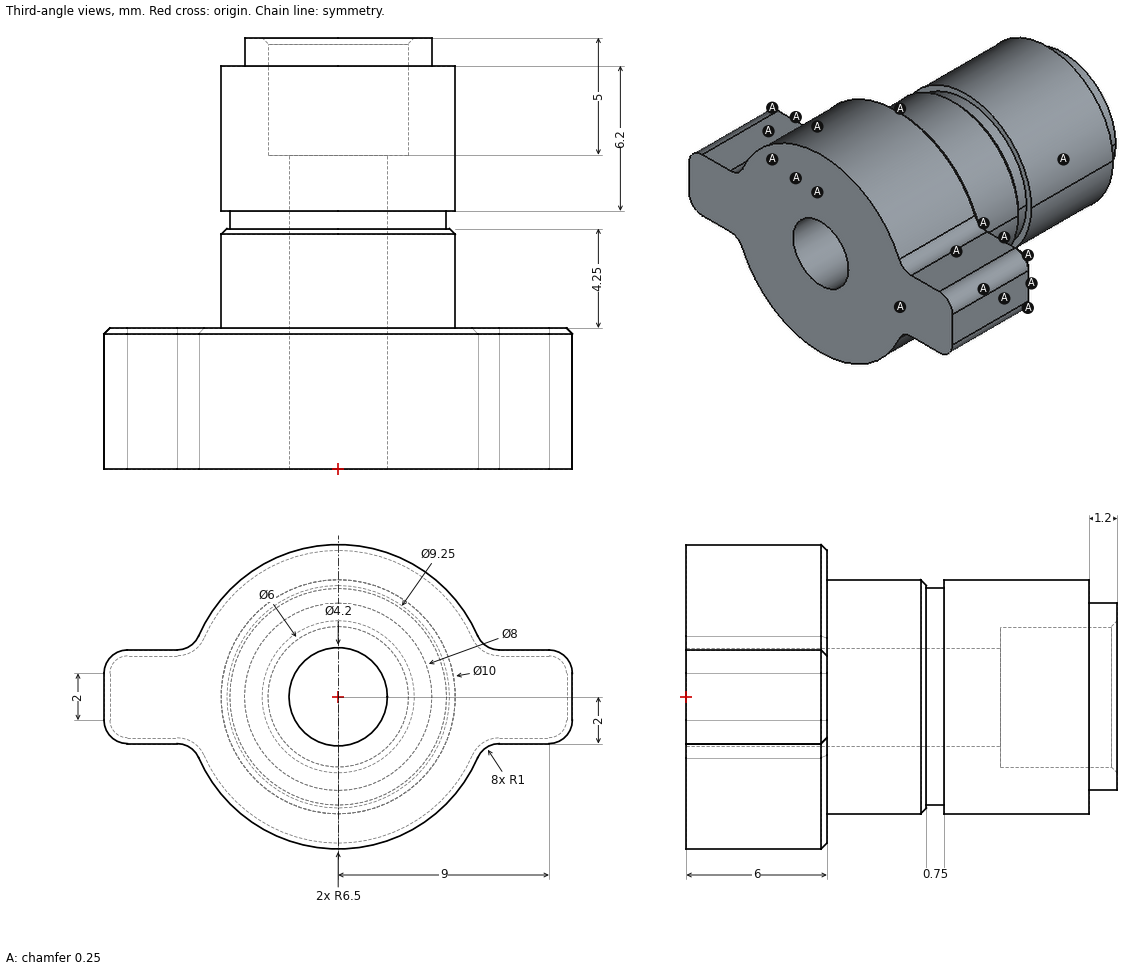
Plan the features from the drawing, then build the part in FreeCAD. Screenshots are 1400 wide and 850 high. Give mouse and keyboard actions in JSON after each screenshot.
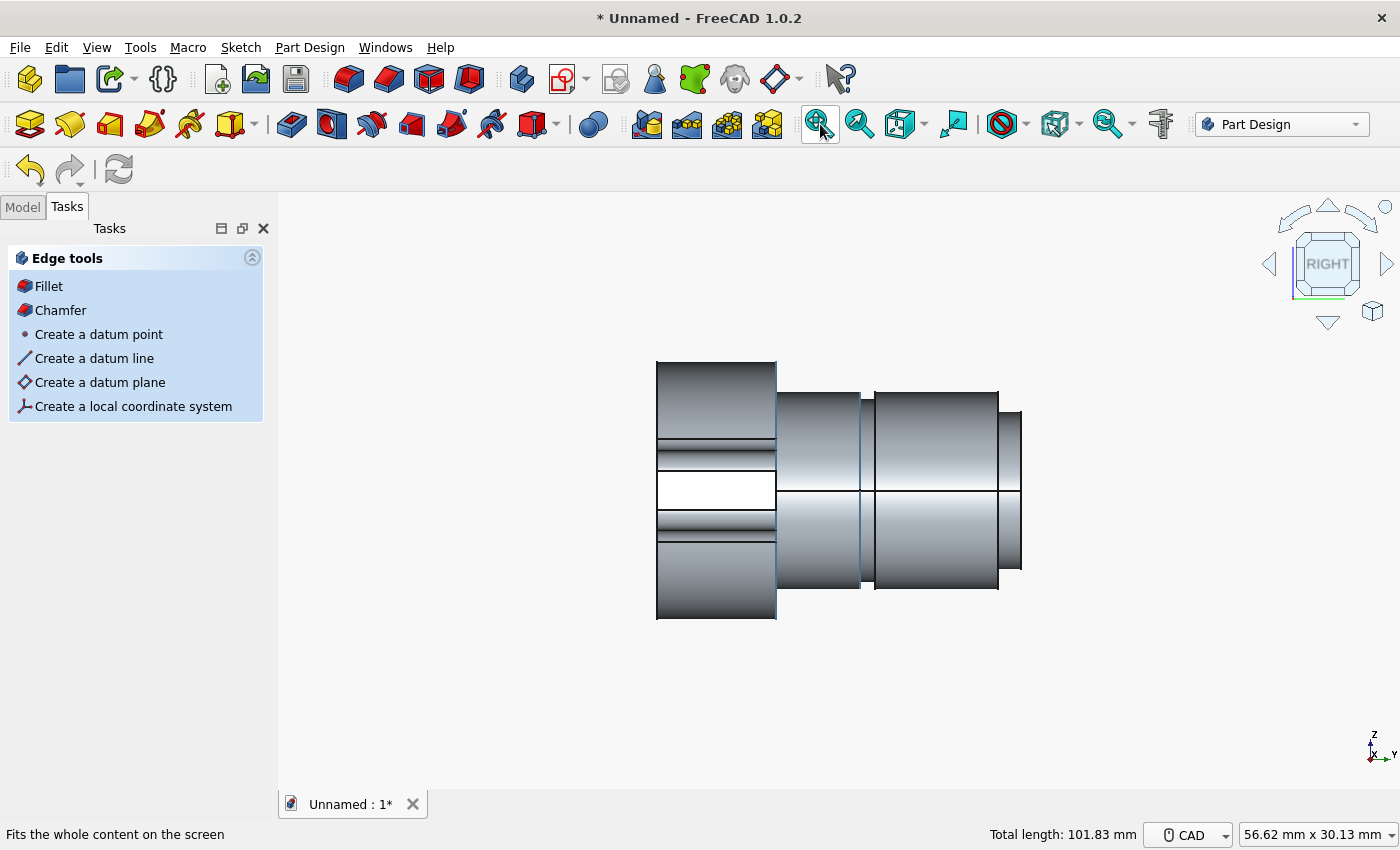
{"action": "left_click", "coordinate": [776, 490], "text": "ctrl"}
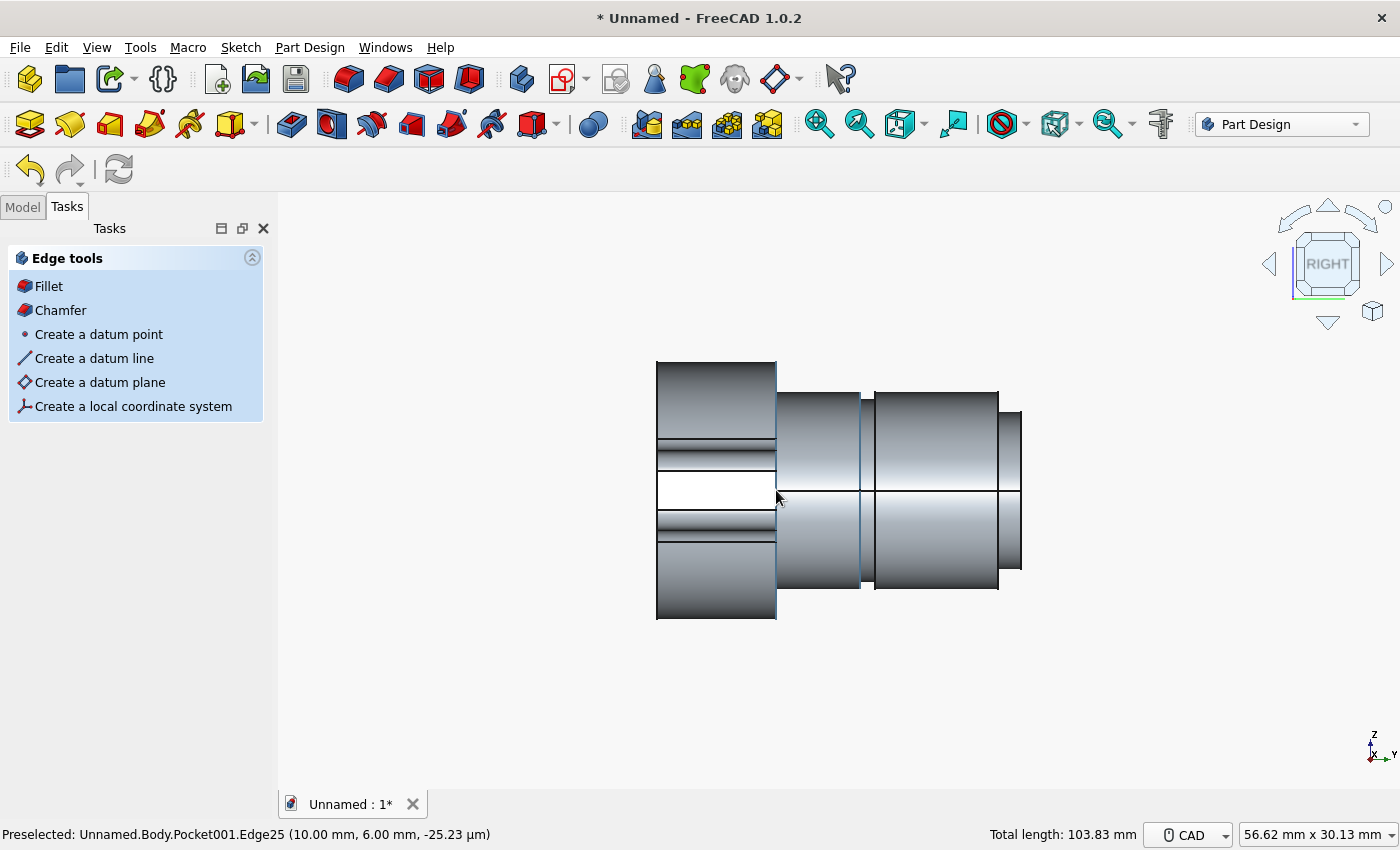
{"action": "left_click", "coordinate": [390, 80]}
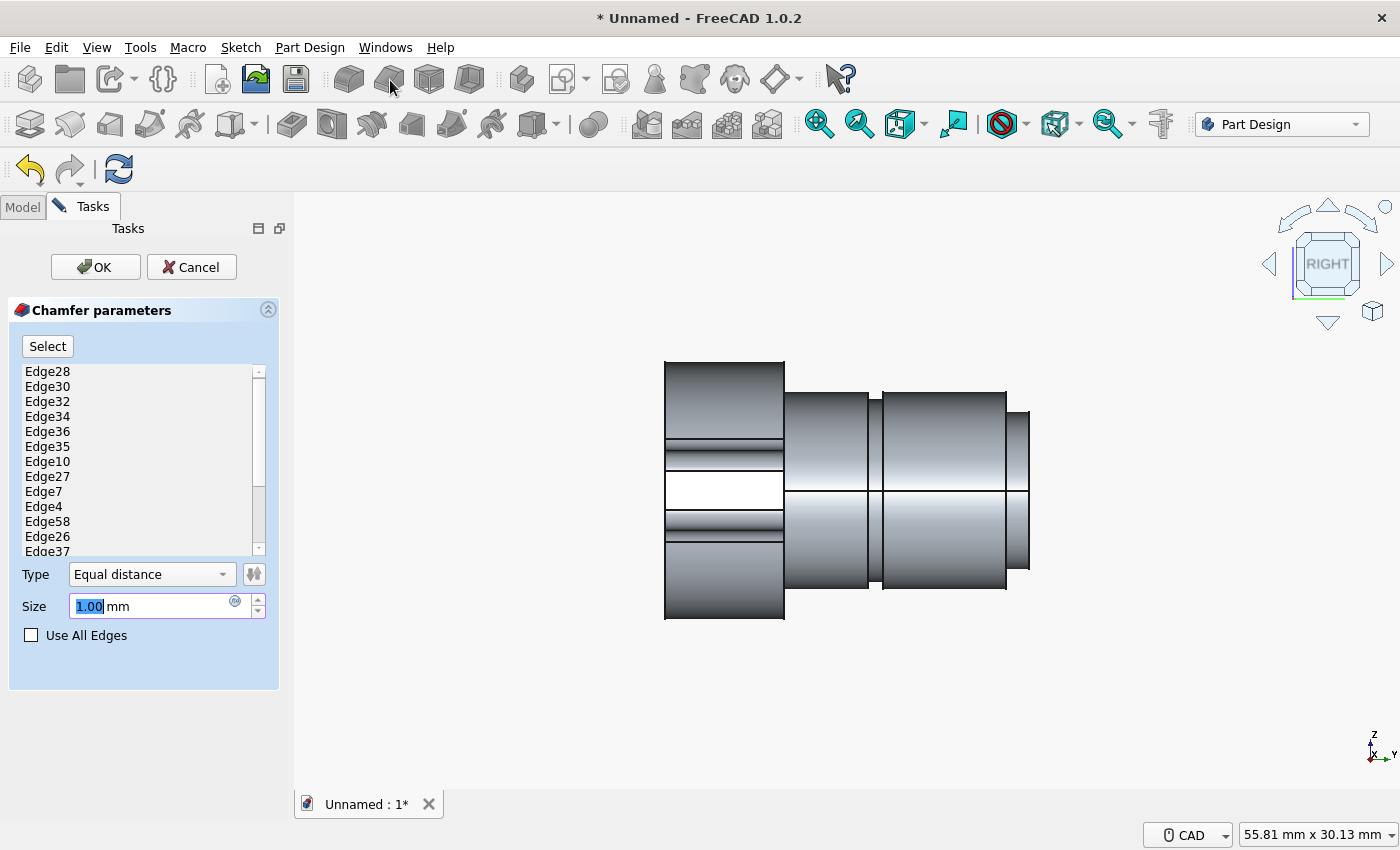
{"action": "type", "text": "0.25"}
{"action": "key", "text": "Tab"}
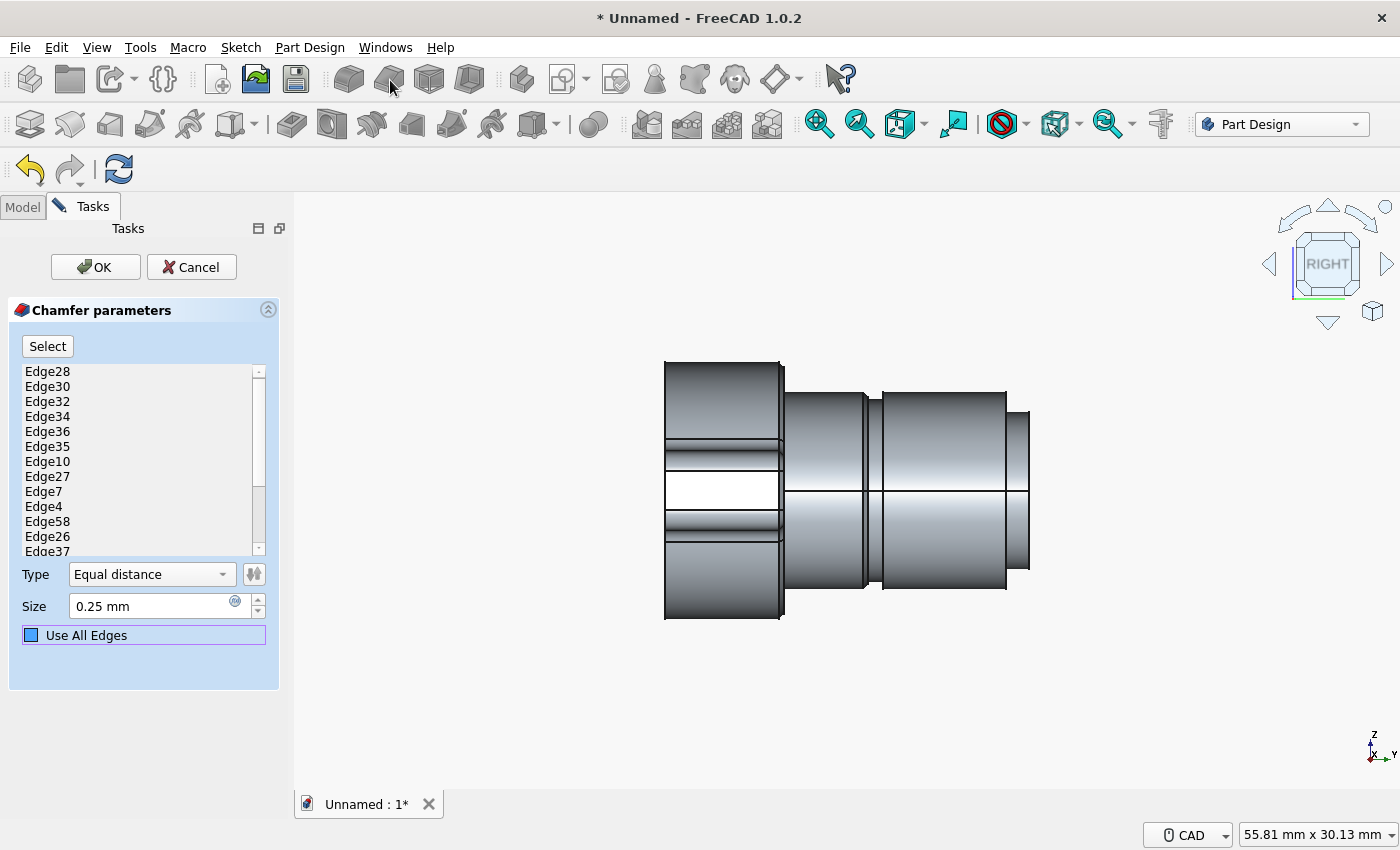
{"action": "left_click", "coordinate": [96, 267]}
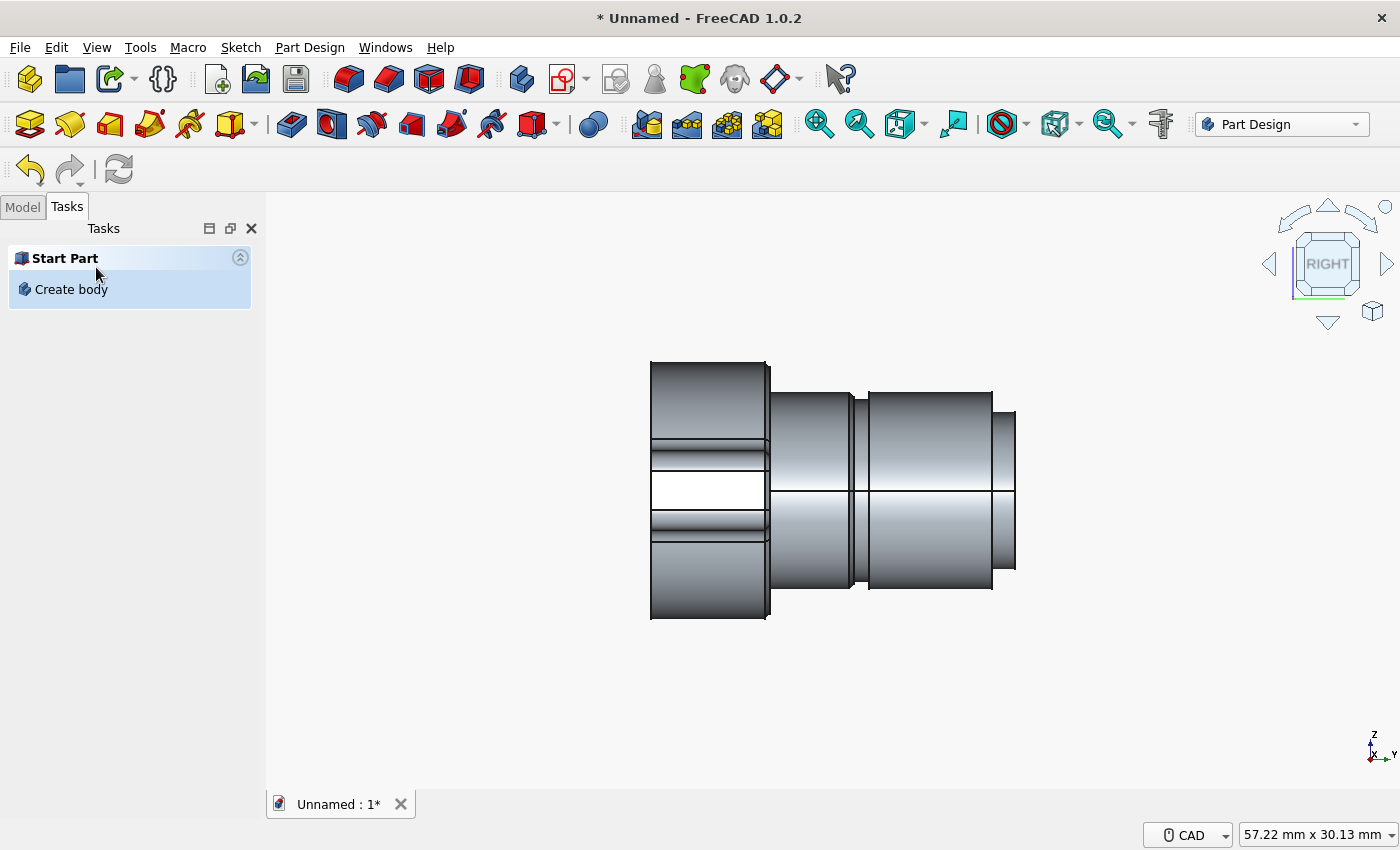
{"action": "key", "text": "0"}